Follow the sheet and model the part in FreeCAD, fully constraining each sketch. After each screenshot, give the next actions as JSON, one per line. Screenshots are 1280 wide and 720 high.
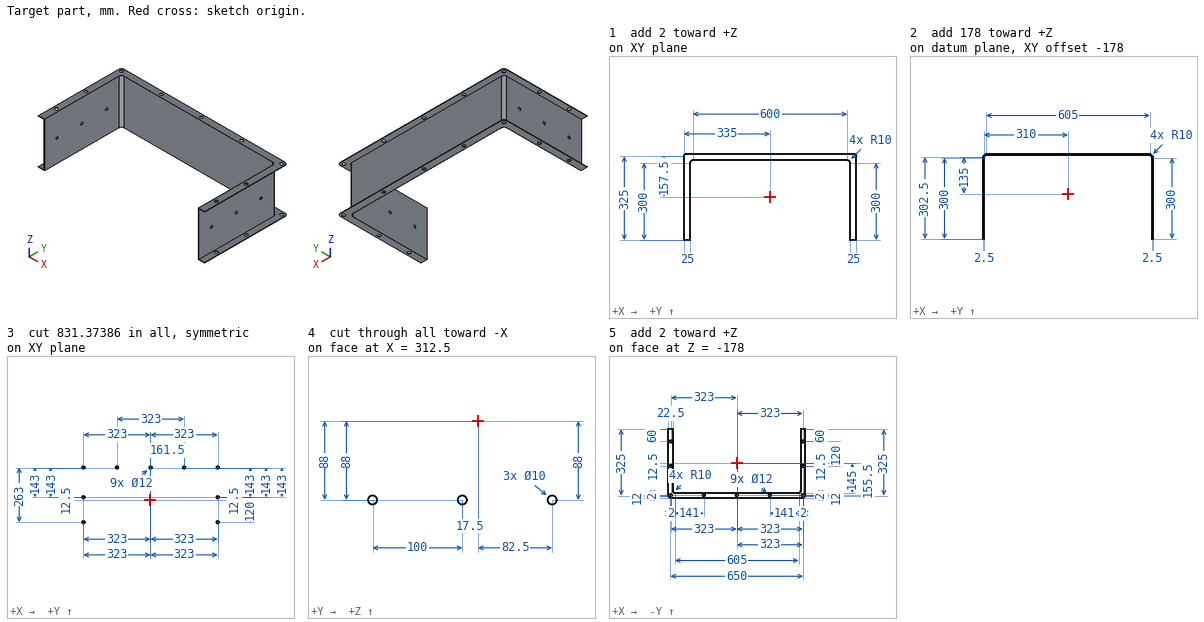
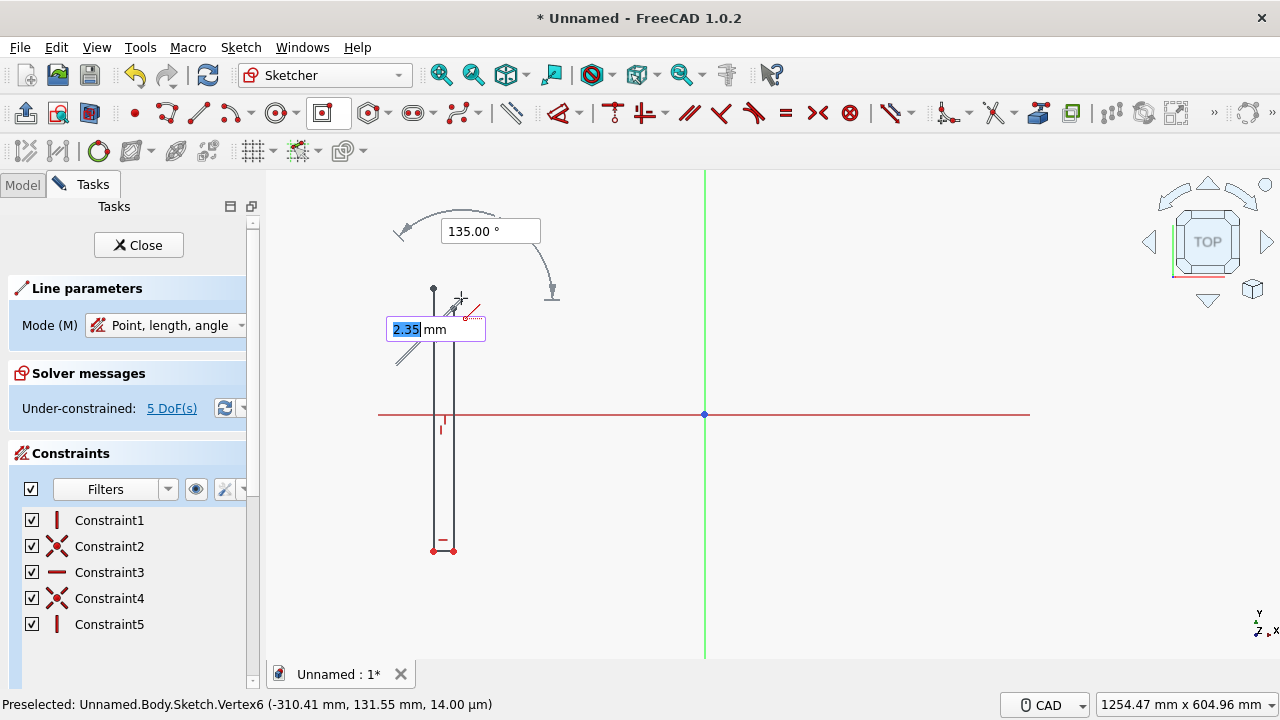
{"action": "left_click", "coordinate": [947, 299]}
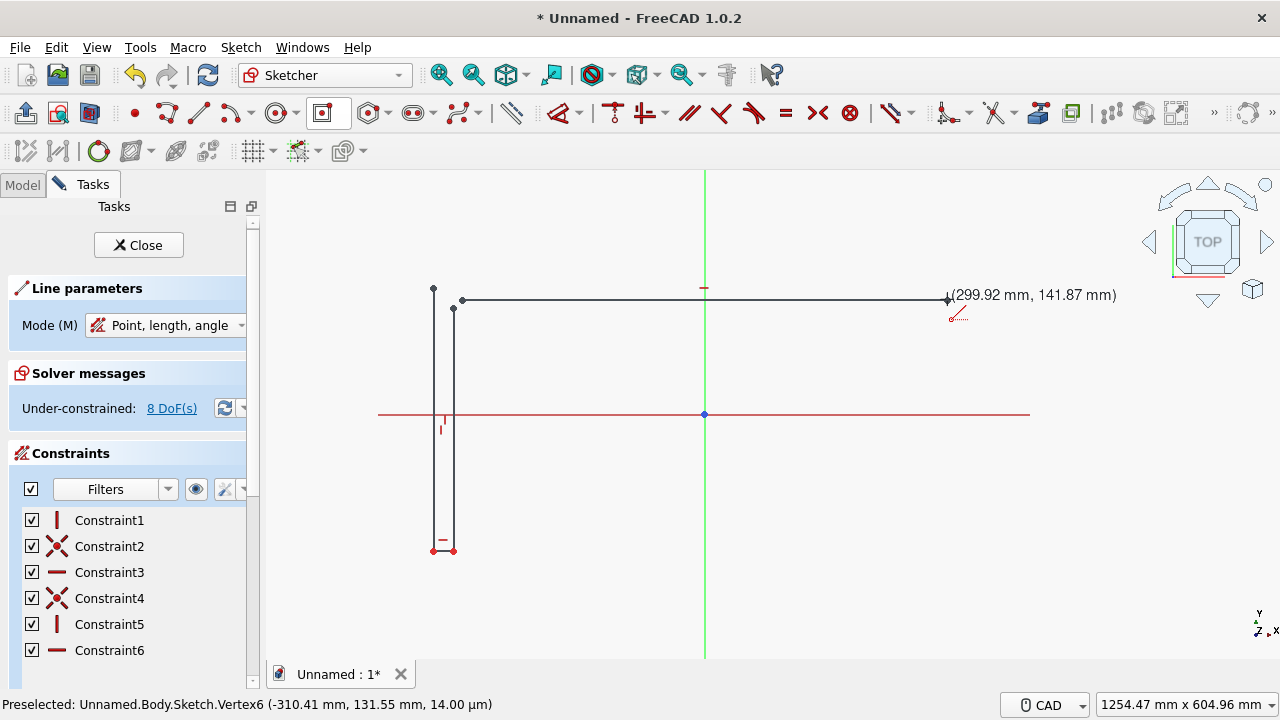
{"action": "key", "text": "g m"}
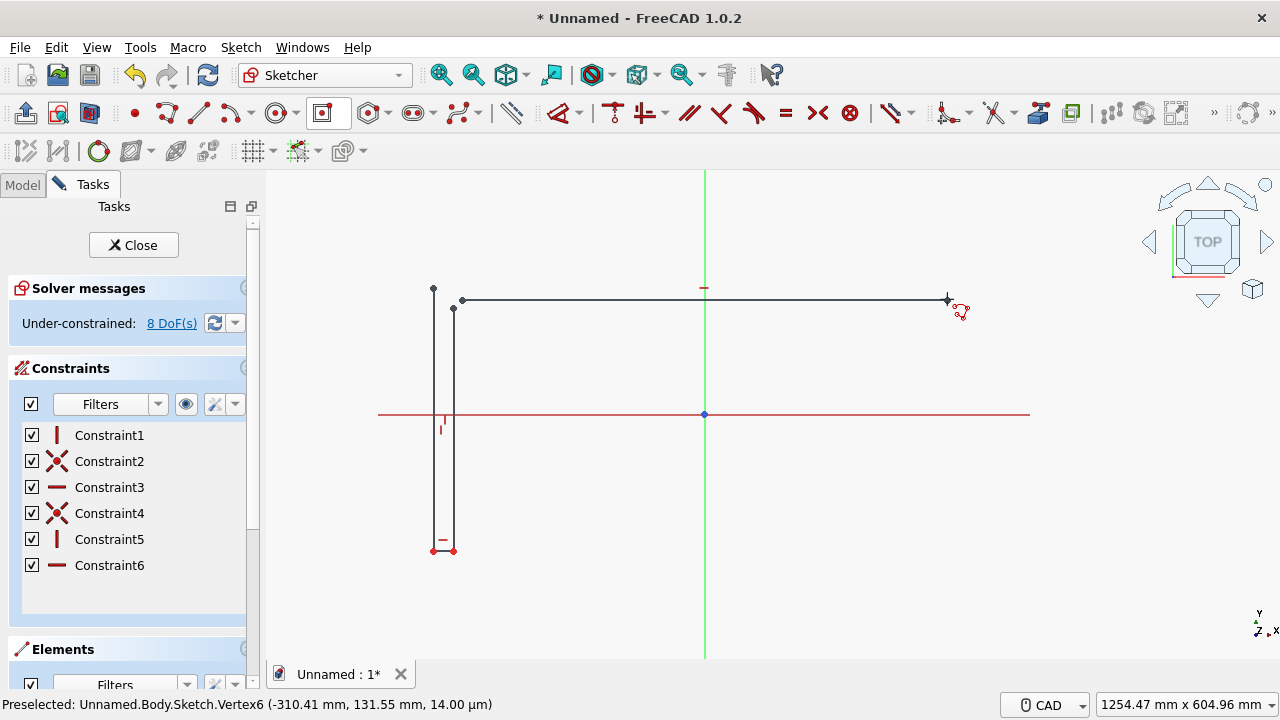
{"action": "scroll", "coordinate": [955, 308], "scroll_direction": "up", "scroll_amount": 2}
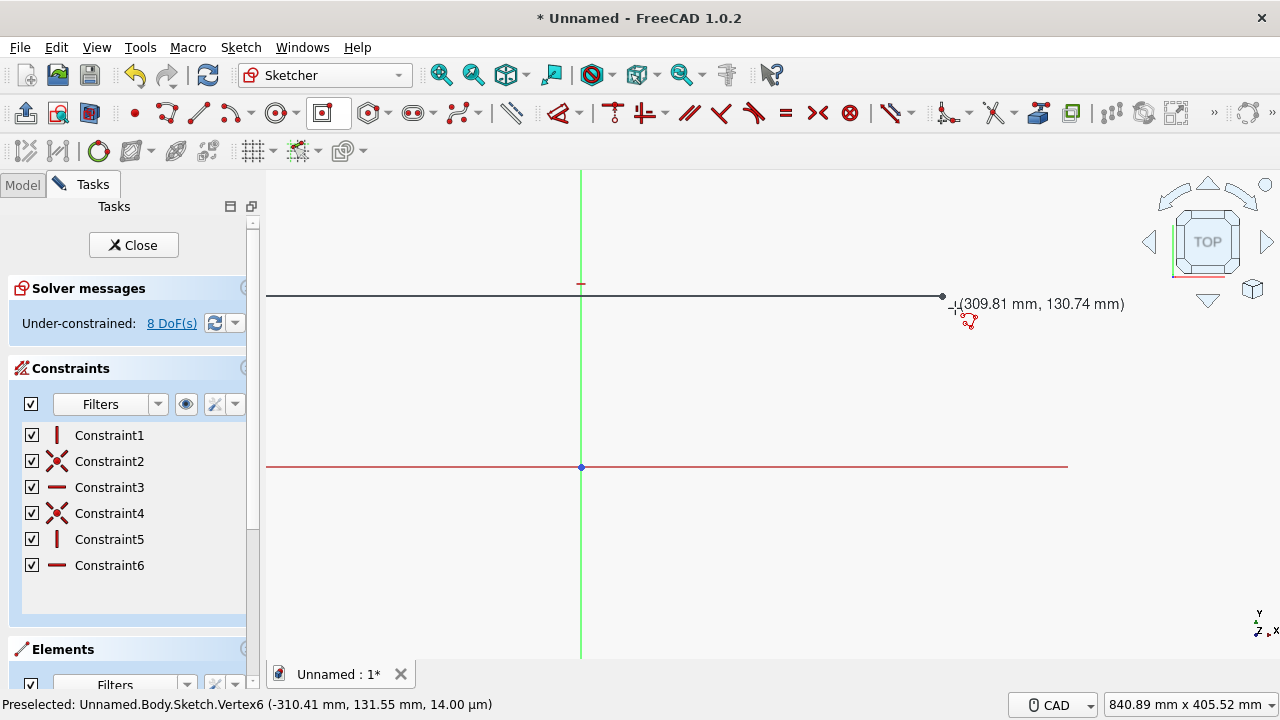
{"action": "left_click", "coordinate": [955, 307]}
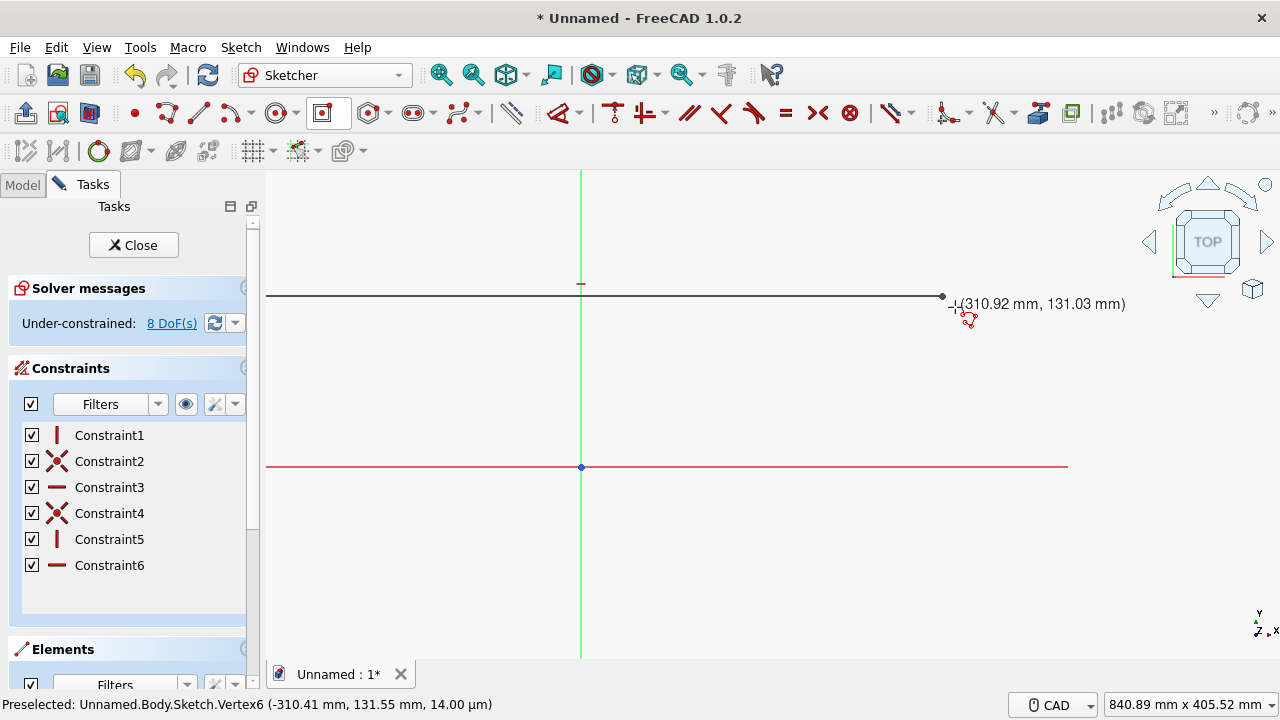
{"action": "scroll", "coordinate": [955, 308], "scroll_direction": "down", "scroll_amount": 2}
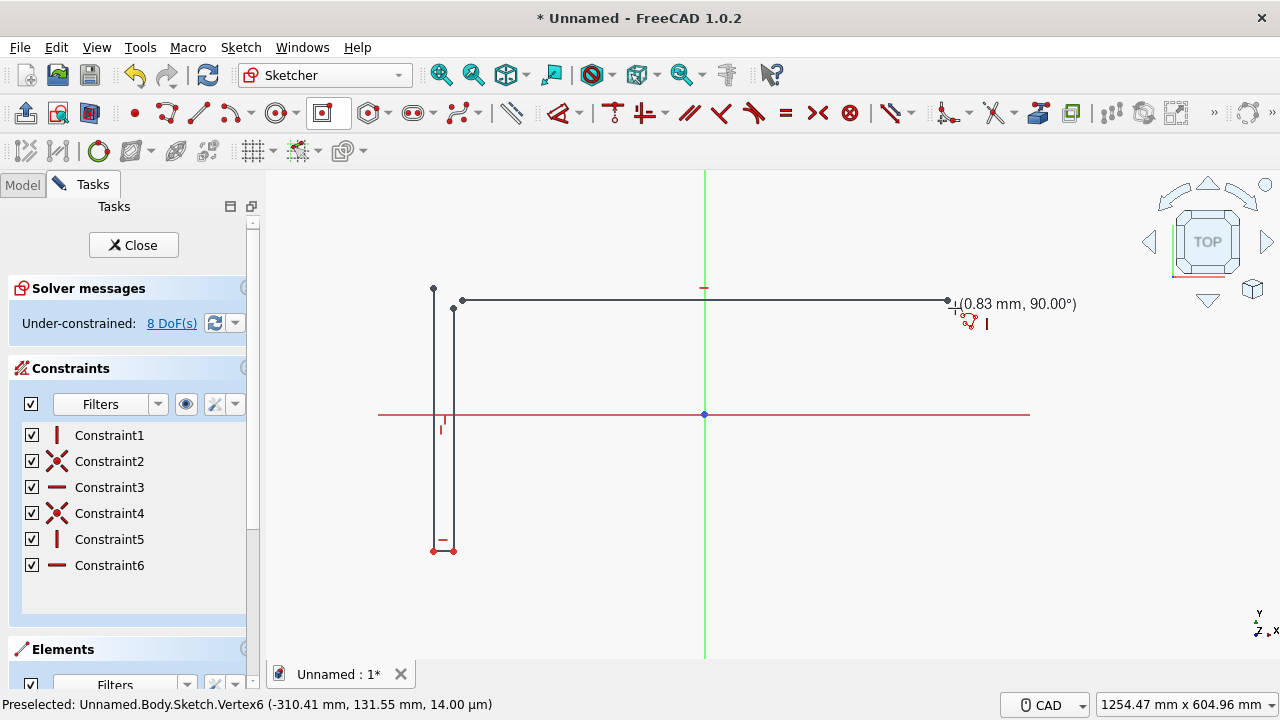
{"action": "left_click", "coordinate": [955, 550]}
{"action": "left_click", "coordinate": [975, 550]}
{"action": "left_click", "coordinate": [975, 287]}
{"action": "right_click", "coordinate": [975, 287]}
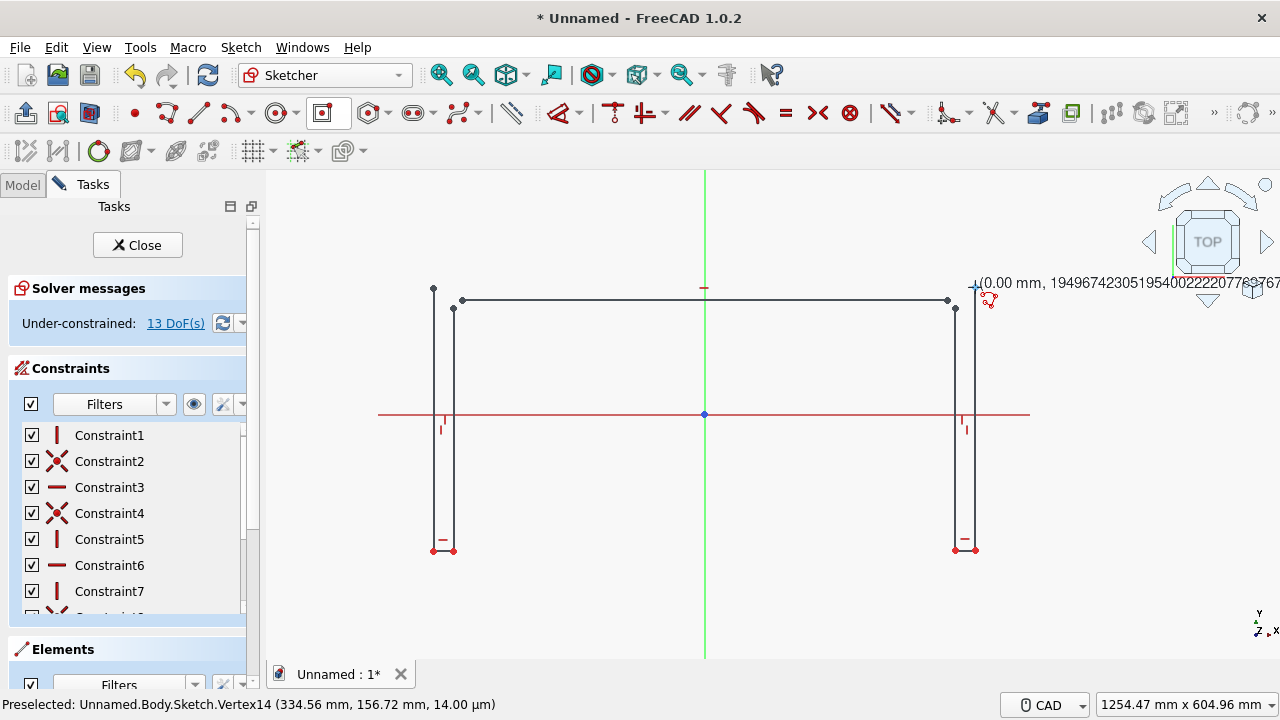
{"action": "left_click", "coordinate": [200, 114]}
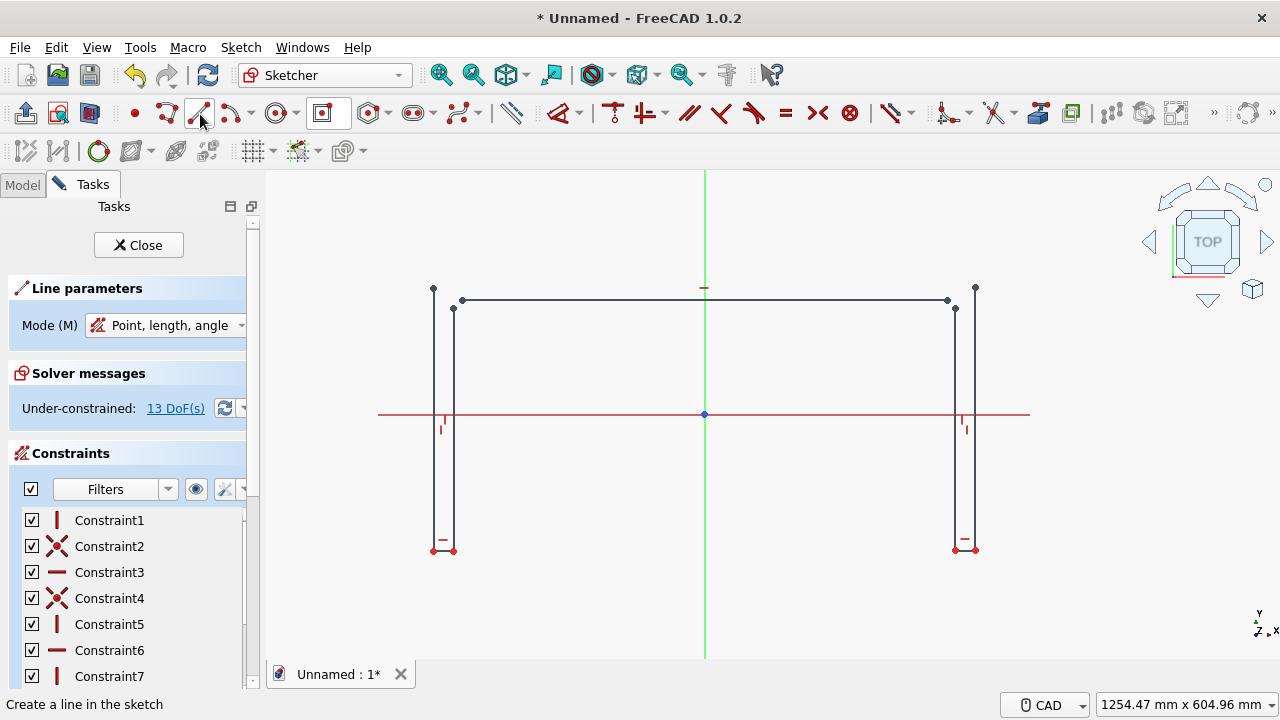
{"action": "scroll", "coordinate": [967, 279], "scroll_direction": "up", "scroll_amount": 2}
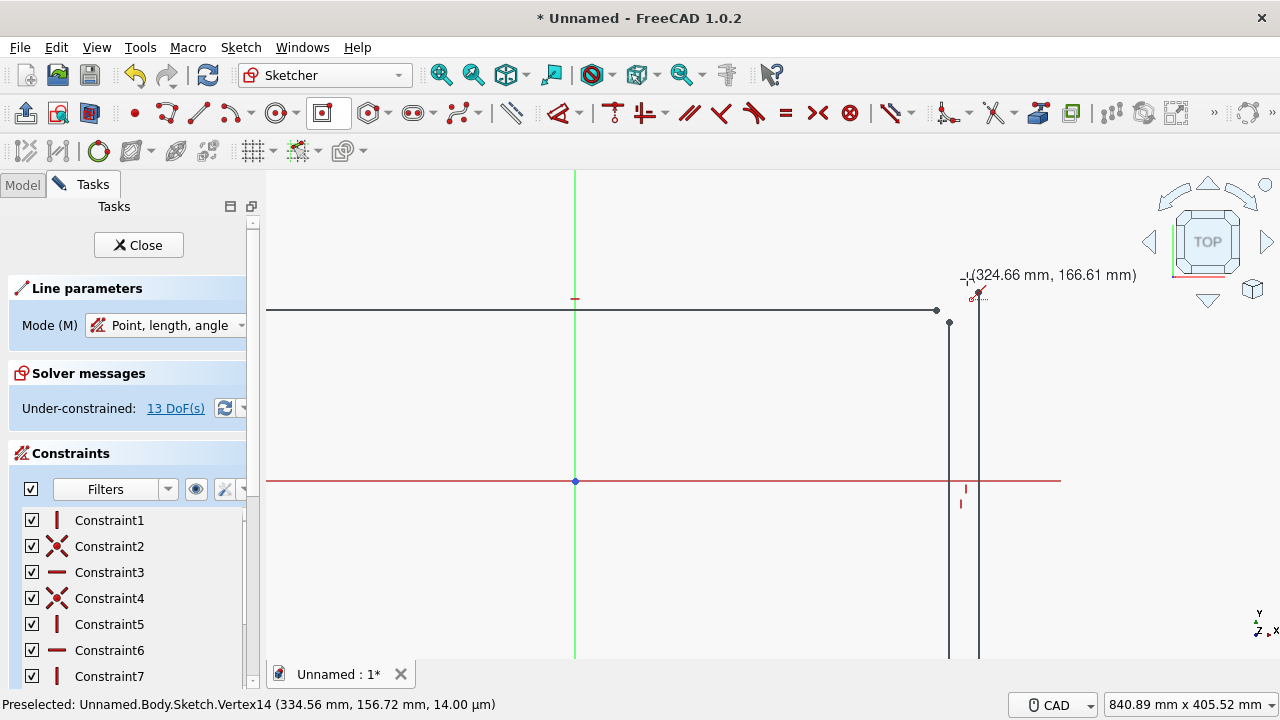
{"action": "left_click", "coordinate": [967, 279]}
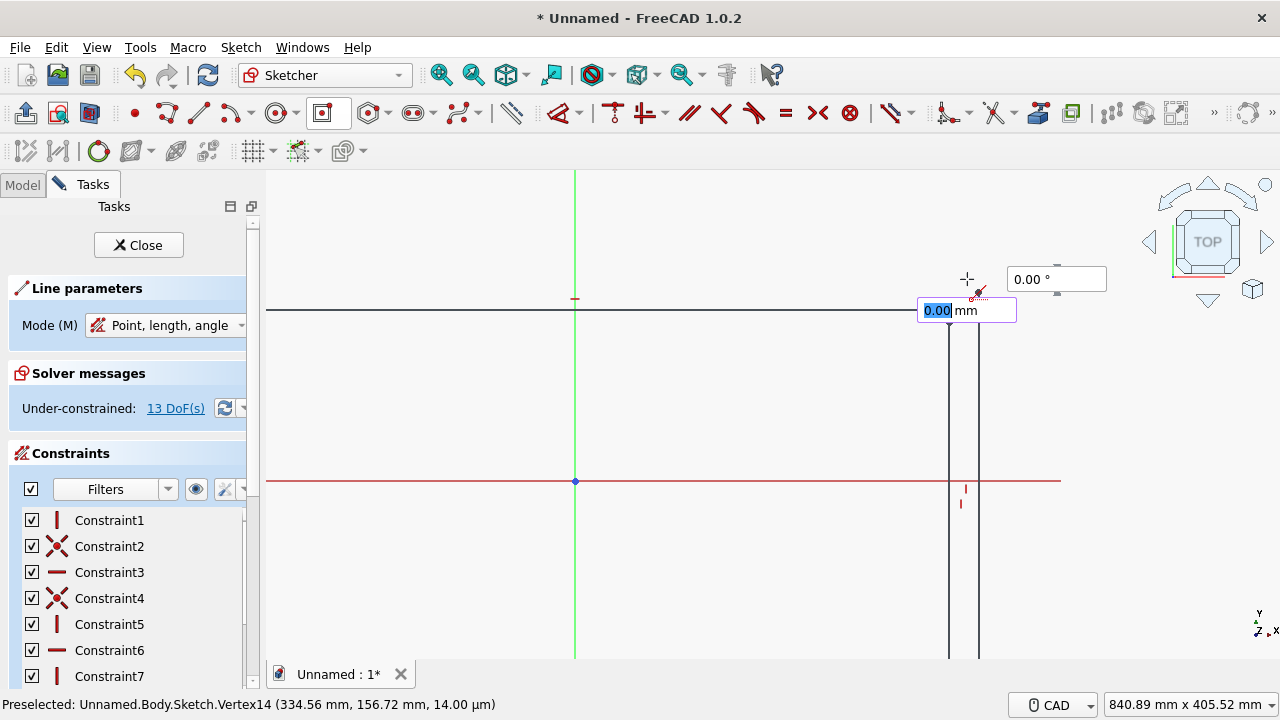
{"action": "scroll", "coordinate": [967, 279], "scroll_direction": "down", "scroll_amount": 2}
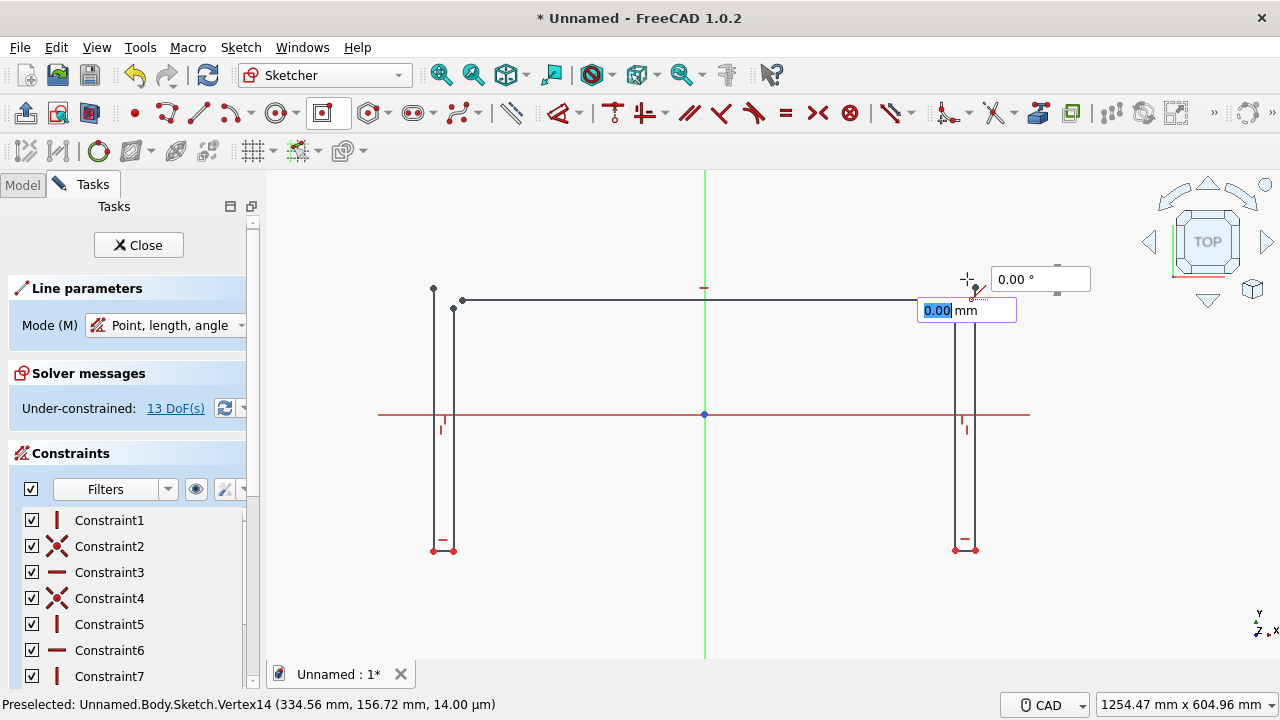
{"action": "scroll", "coordinate": [442, 279], "scroll_direction": "up", "scroll_amount": 2}